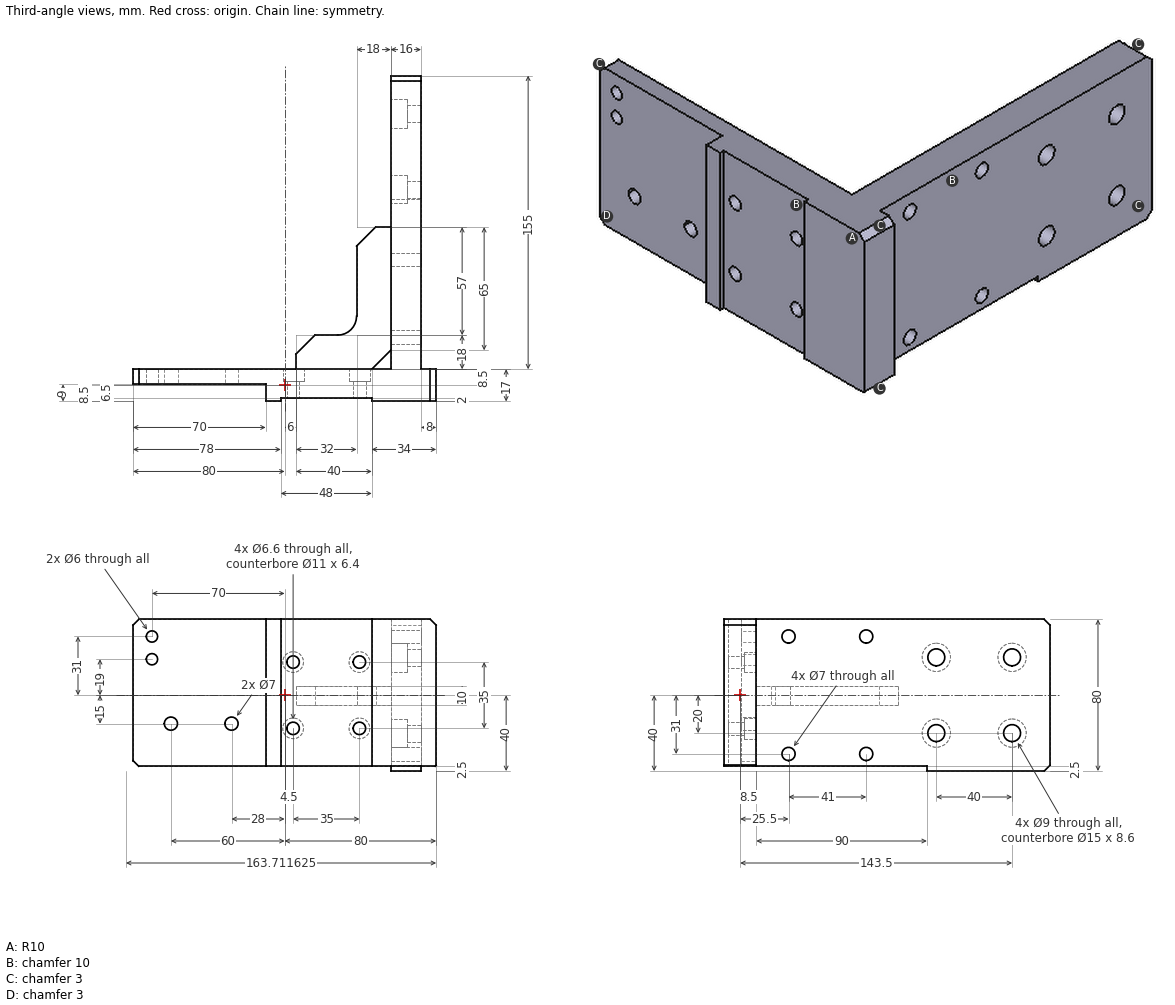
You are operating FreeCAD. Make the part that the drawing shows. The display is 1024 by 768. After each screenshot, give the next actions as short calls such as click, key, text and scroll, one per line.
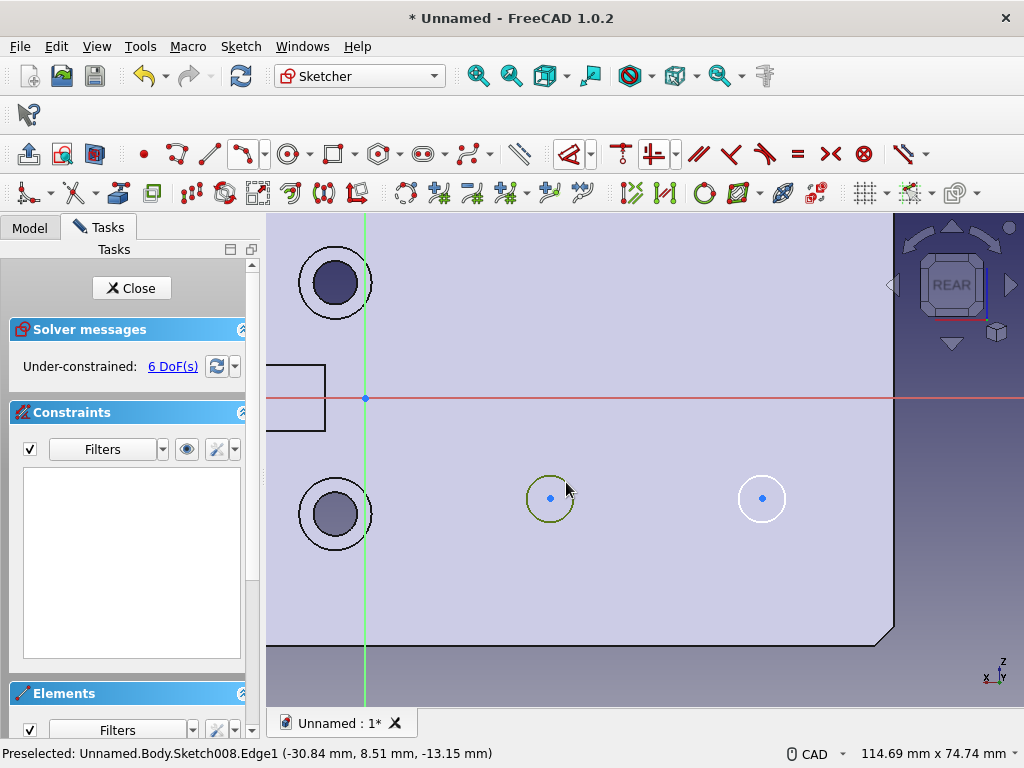
click(778, 482)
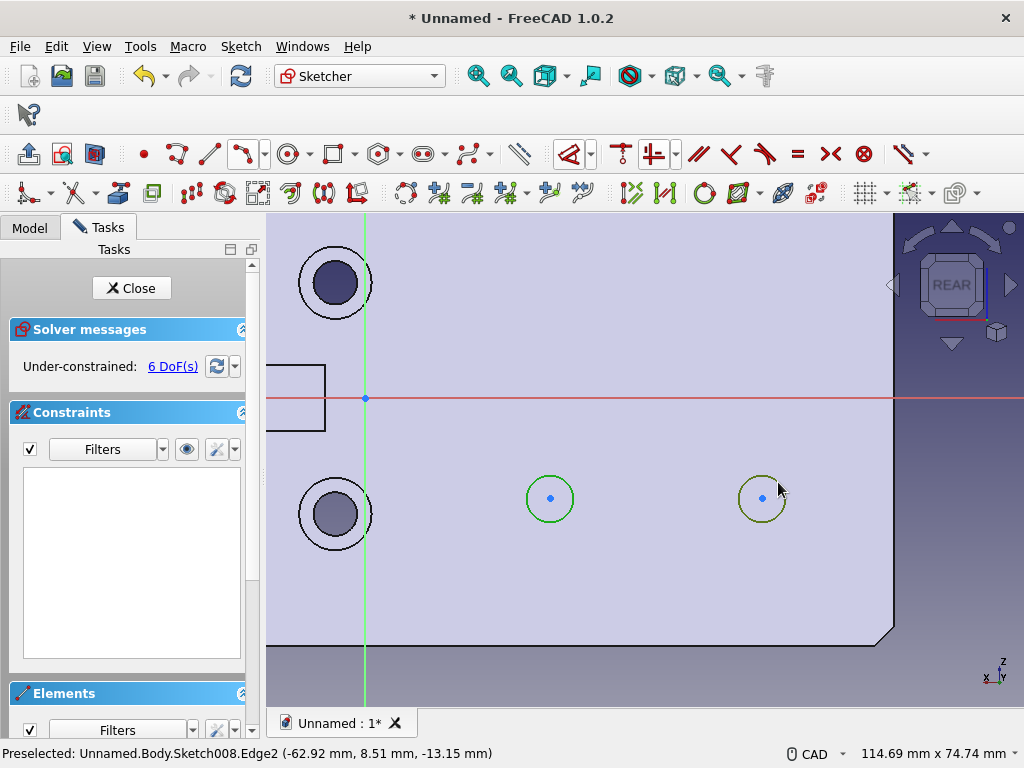
key(e)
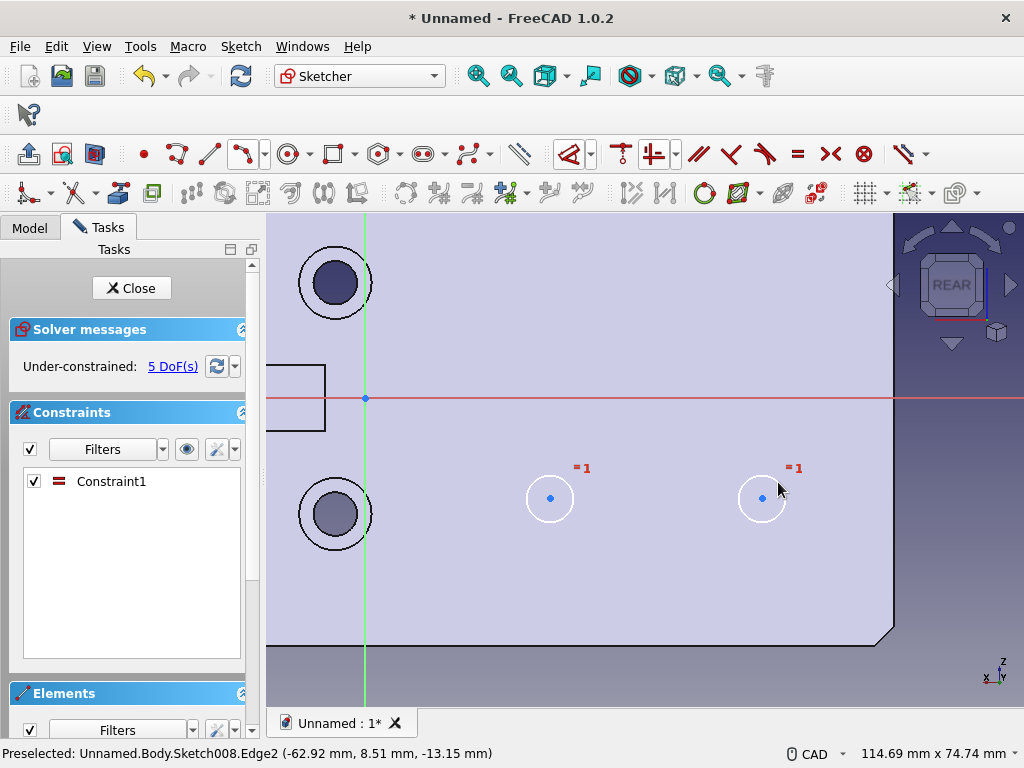
click(566, 482)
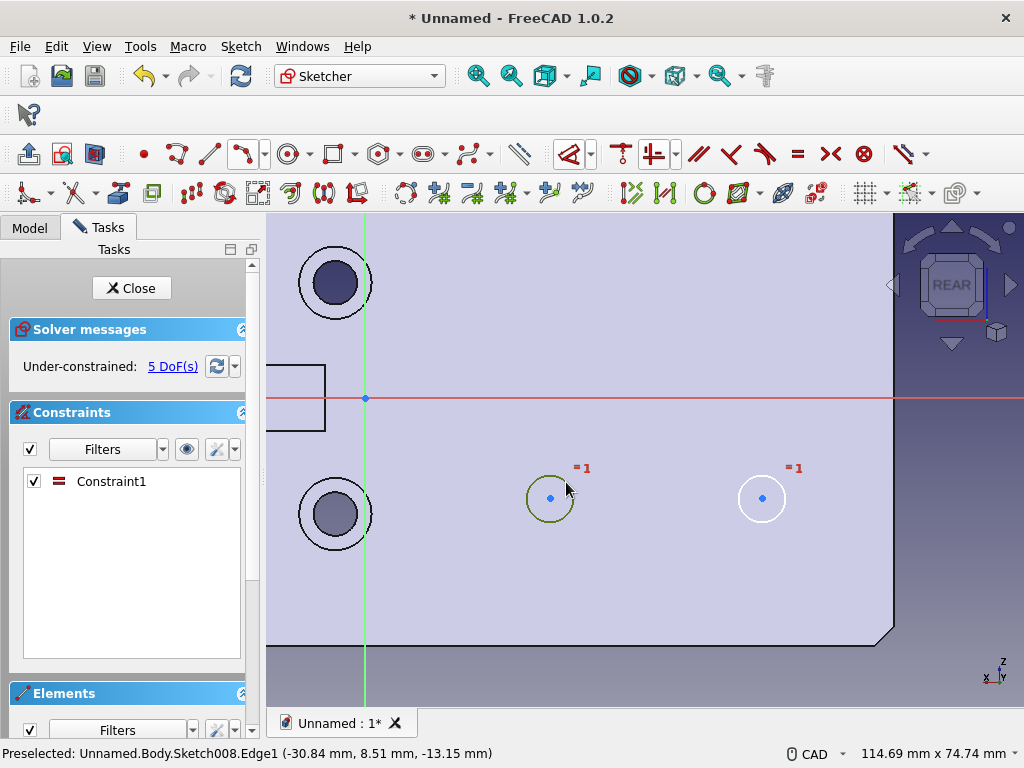
key(k)
key(o)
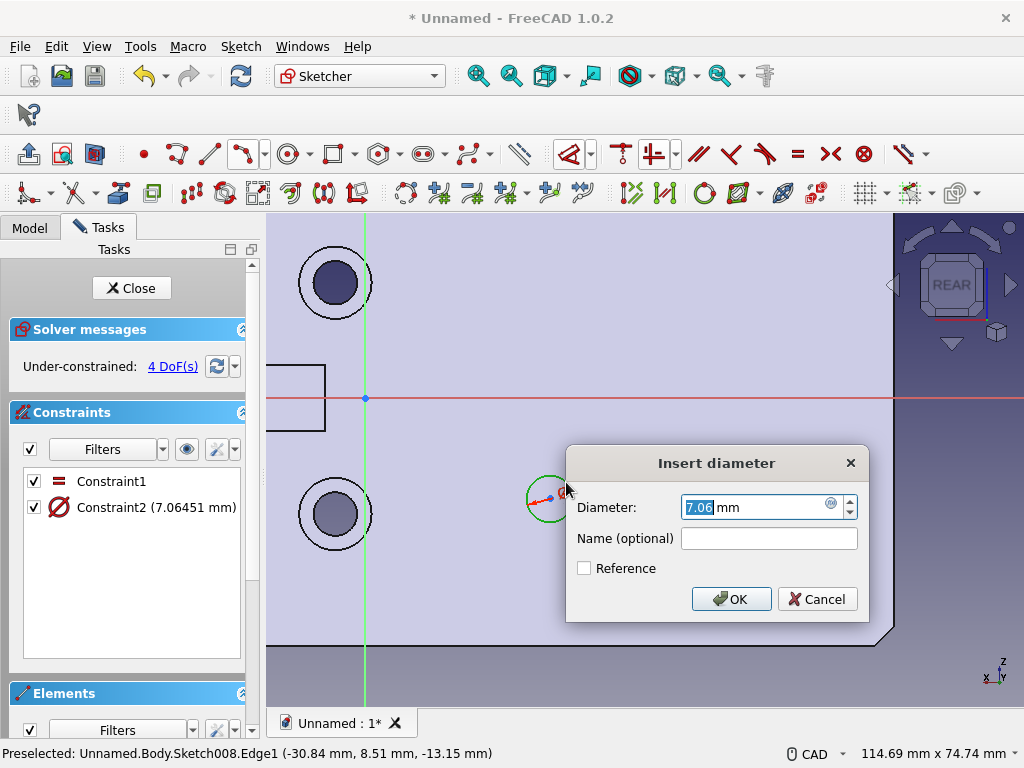
text(7)
key(Return)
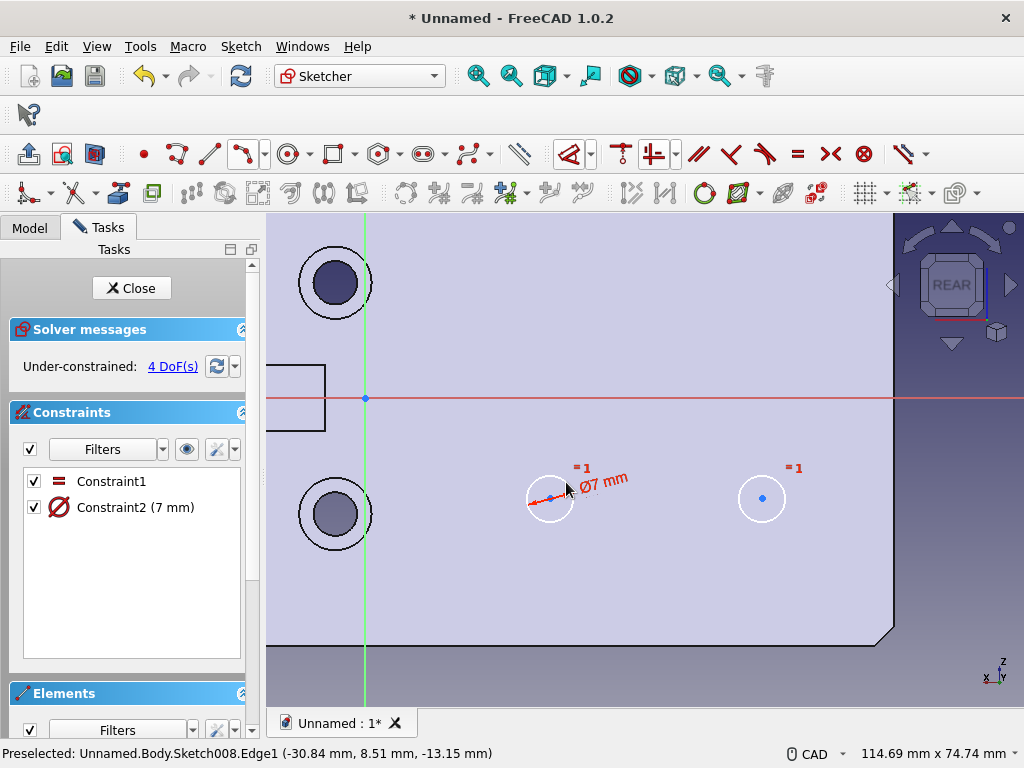
click(550, 499)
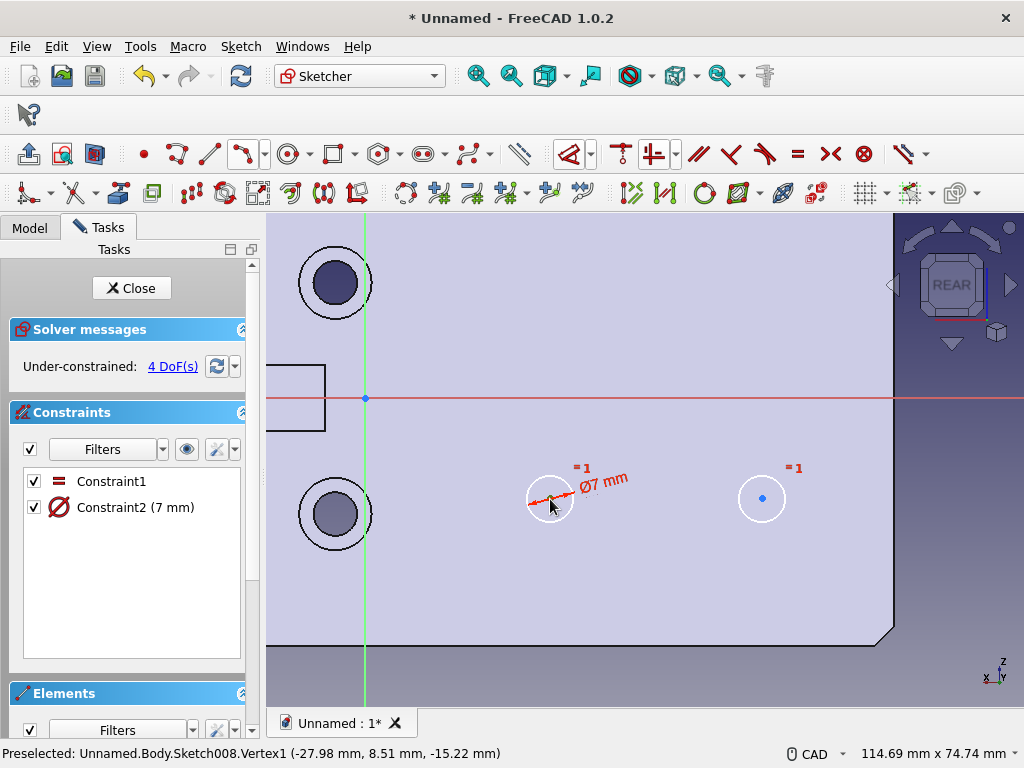
key(l)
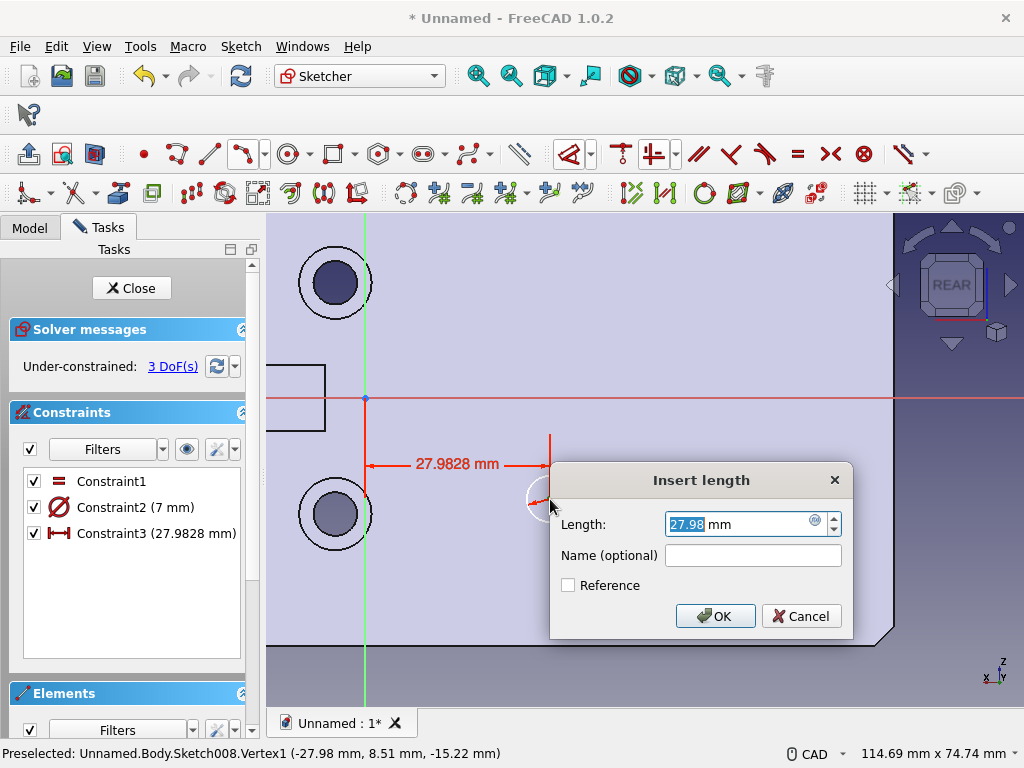
text(28)
key(Return)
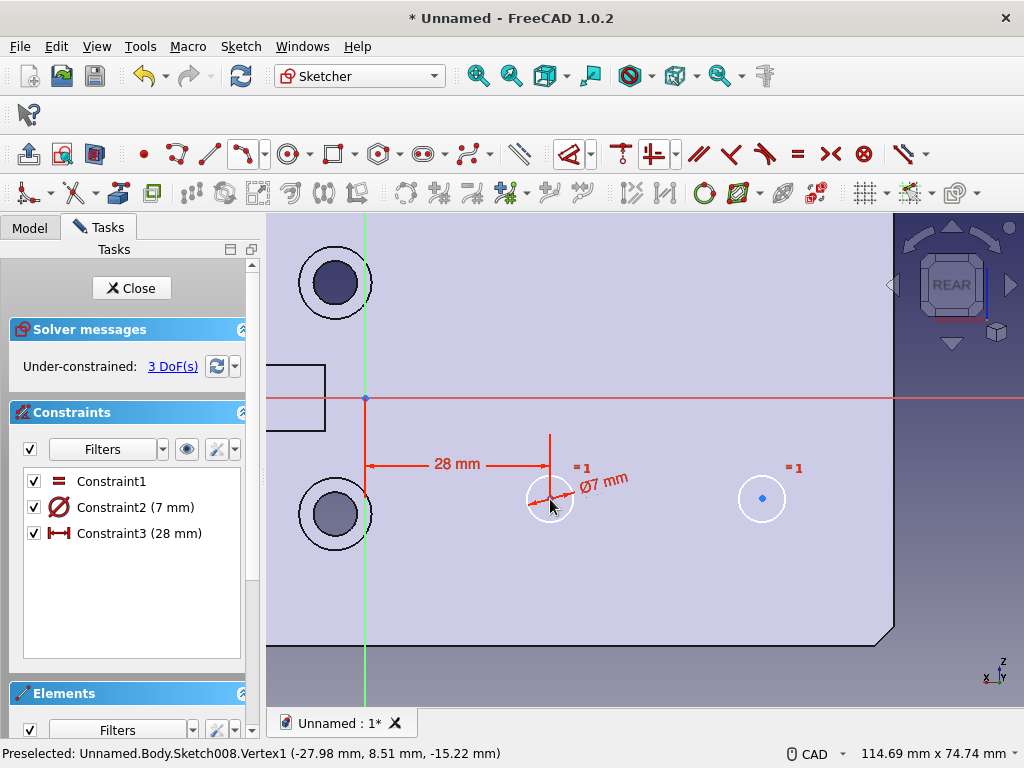
click(550, 499)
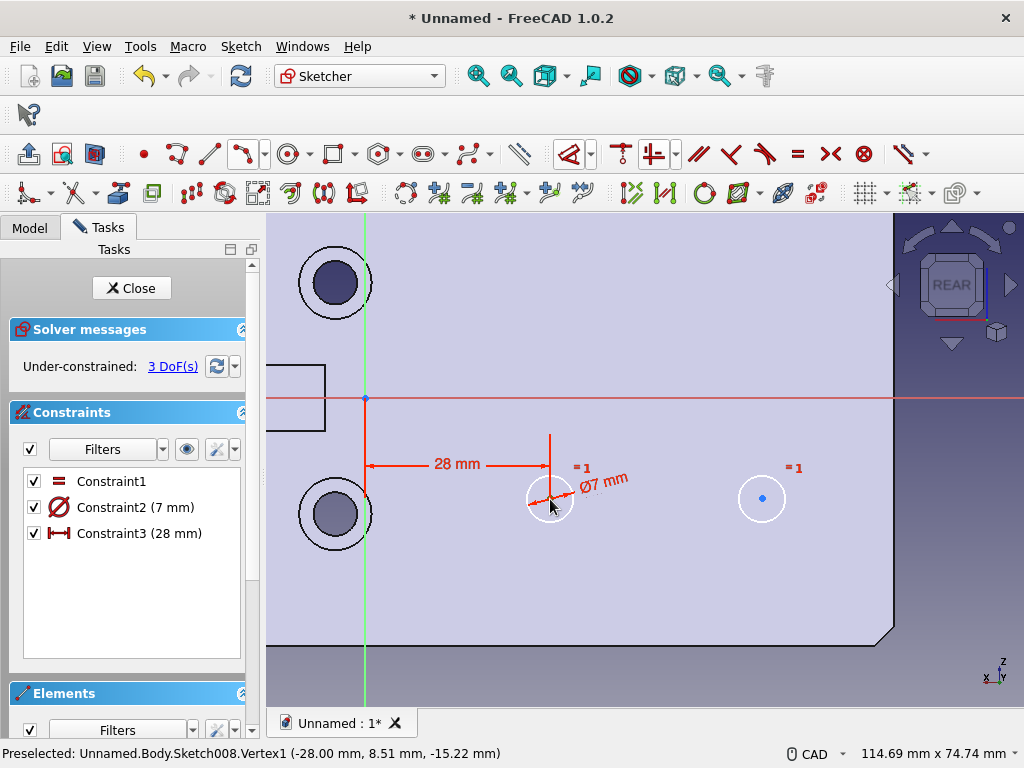
click(590, 154)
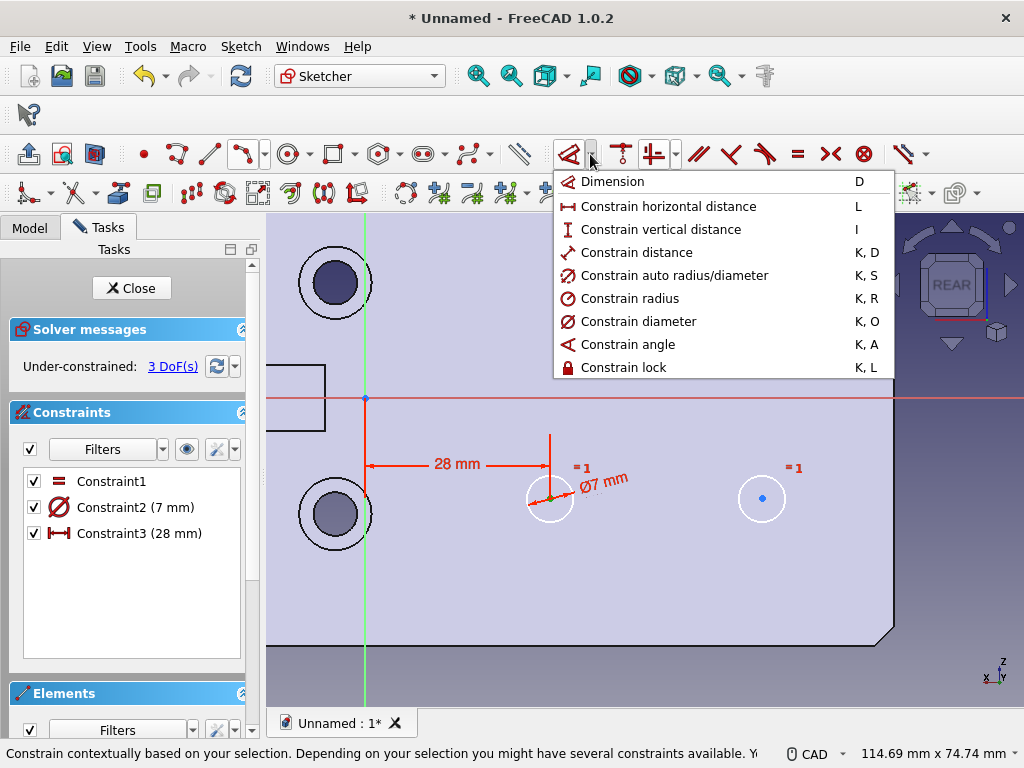
click(724, 230)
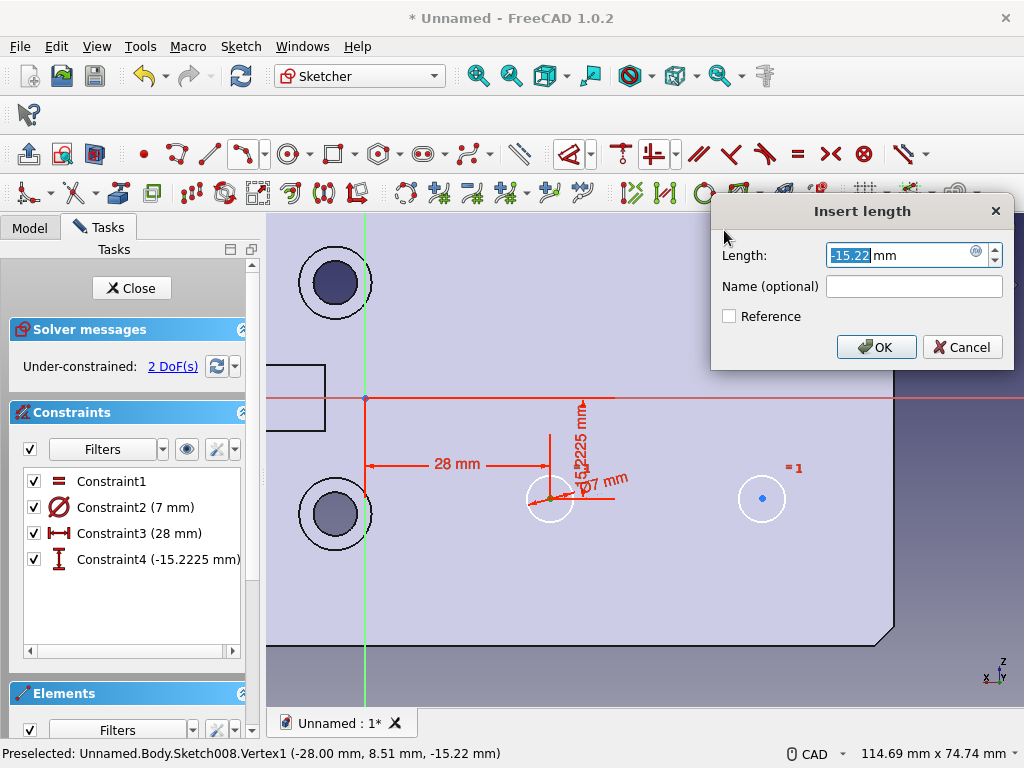
text(-15)
key(Return)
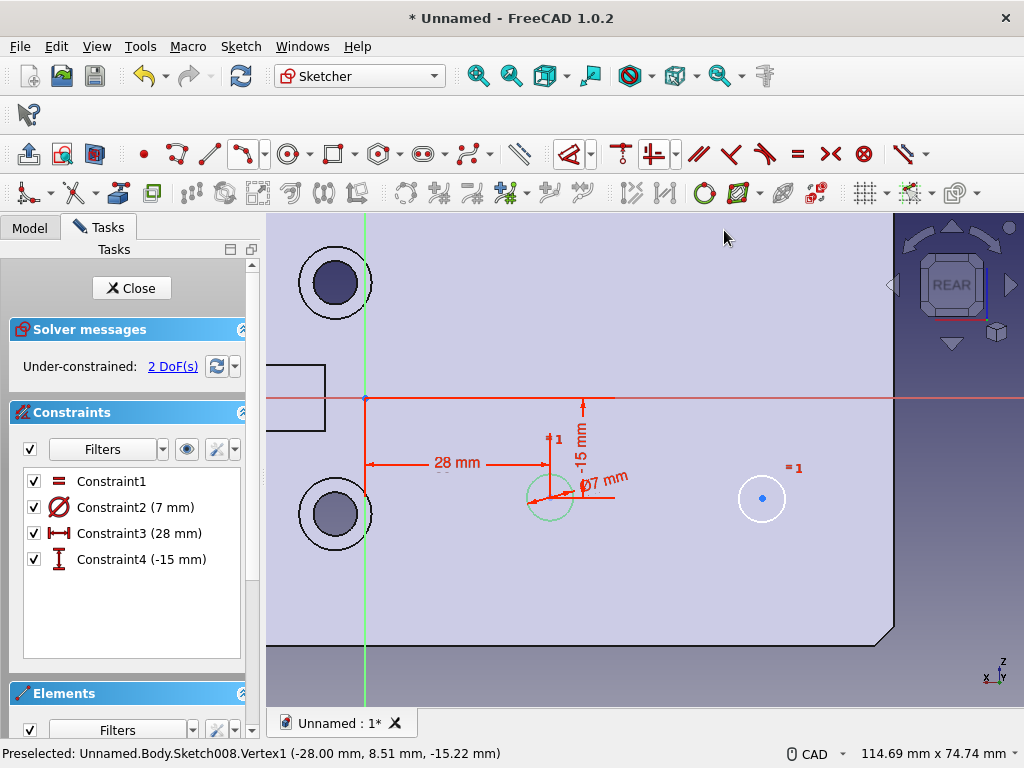
click(762, 499)